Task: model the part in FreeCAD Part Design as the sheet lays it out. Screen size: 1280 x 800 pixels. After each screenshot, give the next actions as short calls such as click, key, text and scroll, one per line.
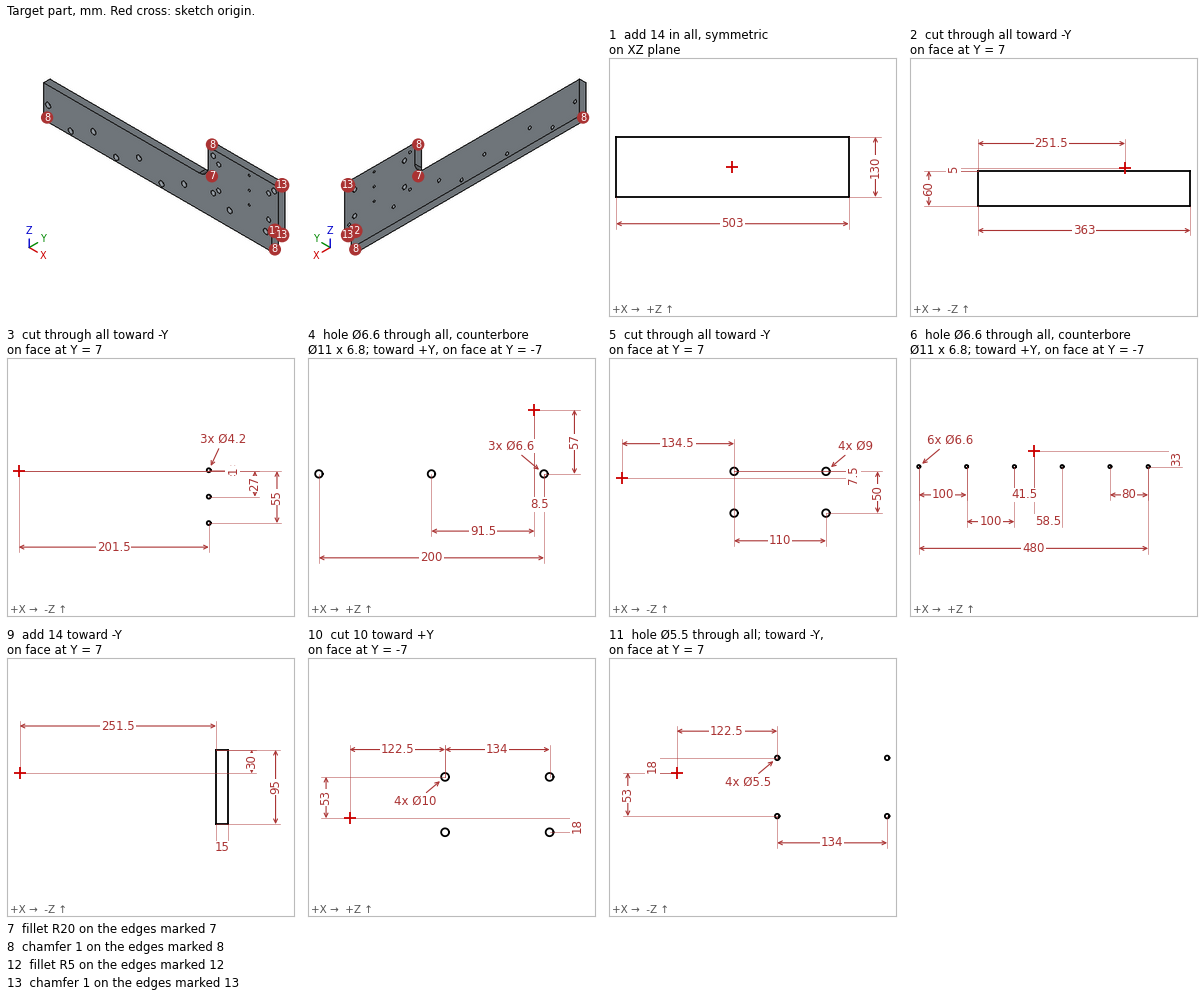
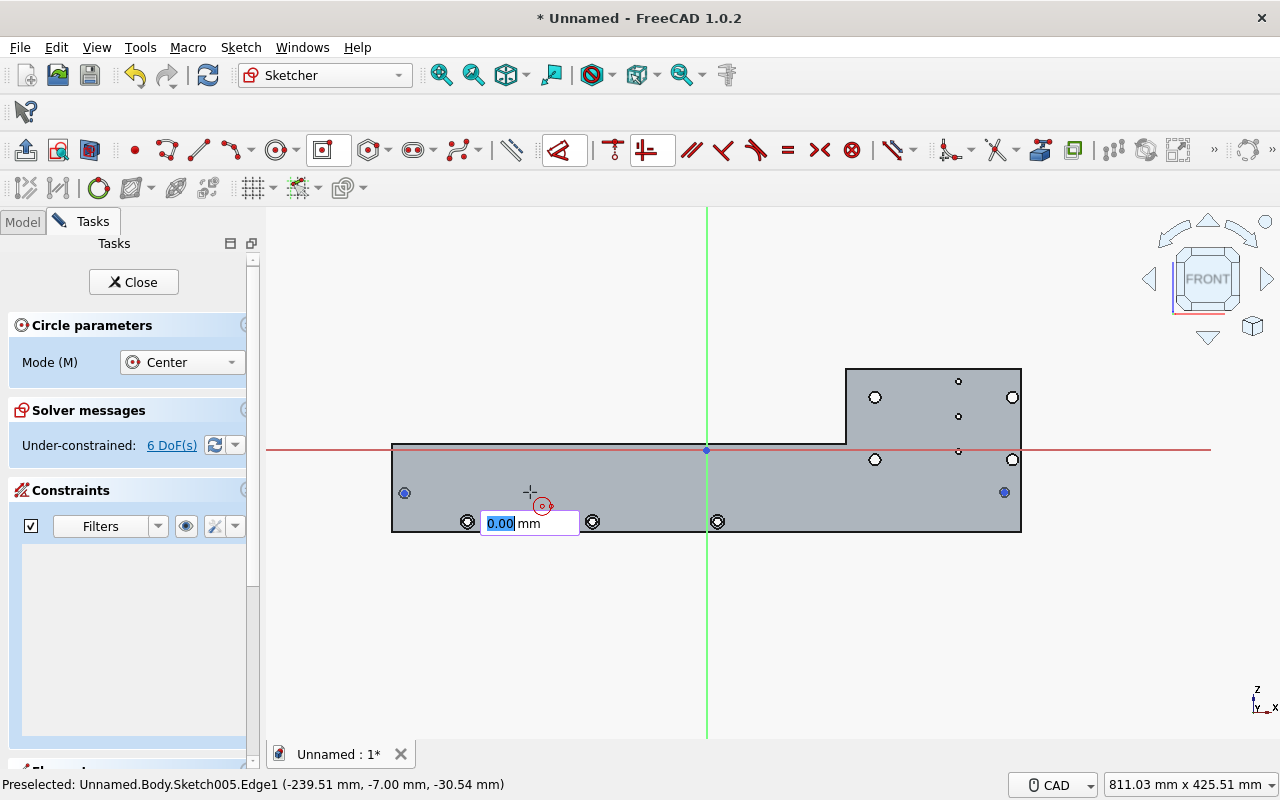
scroll(533, 489, up, 7)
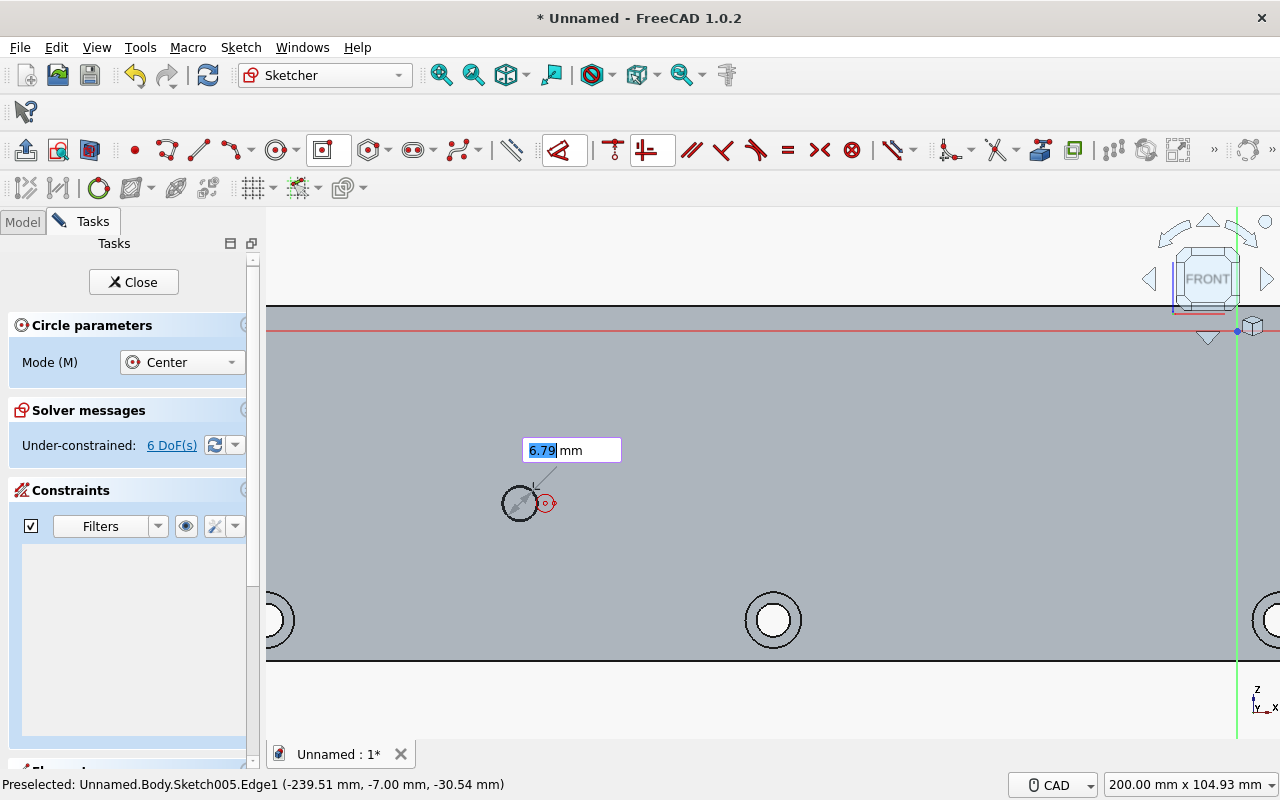
click(532, 487)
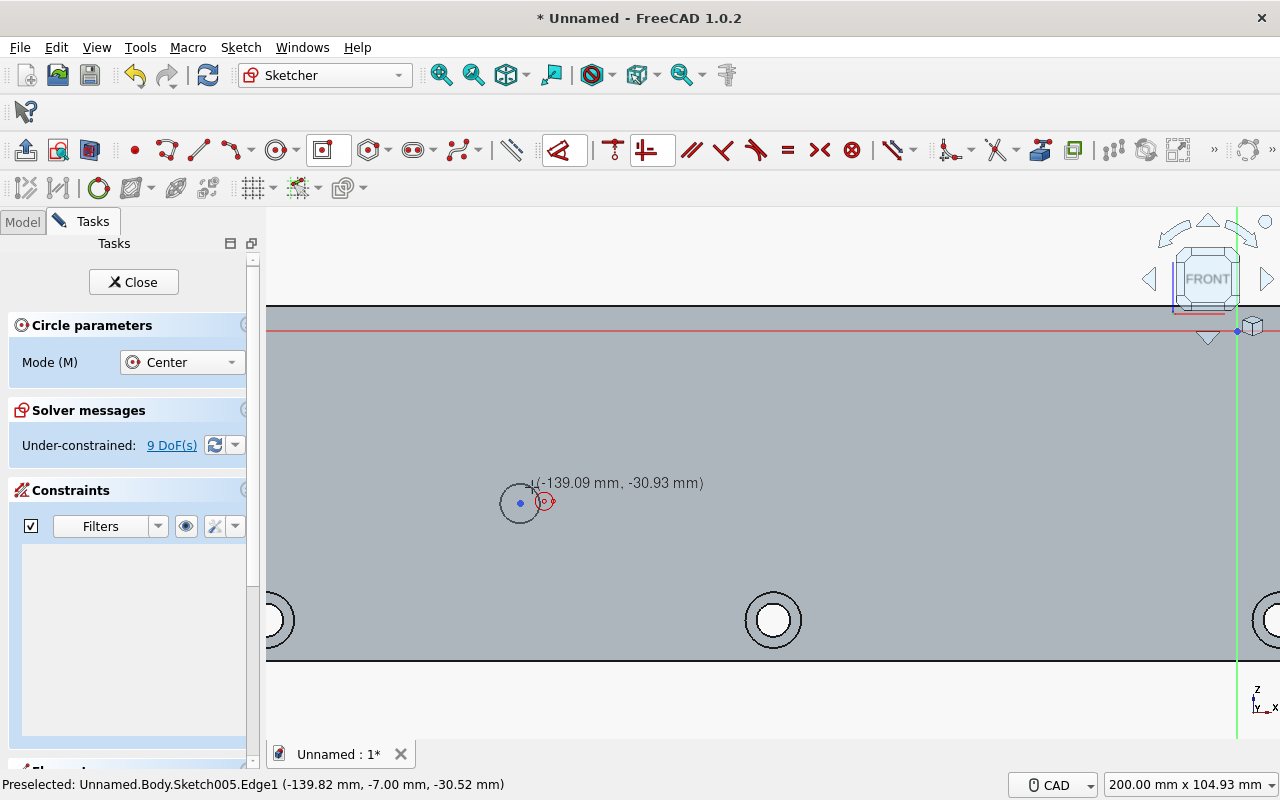
scroll(1027, 498, up, 2)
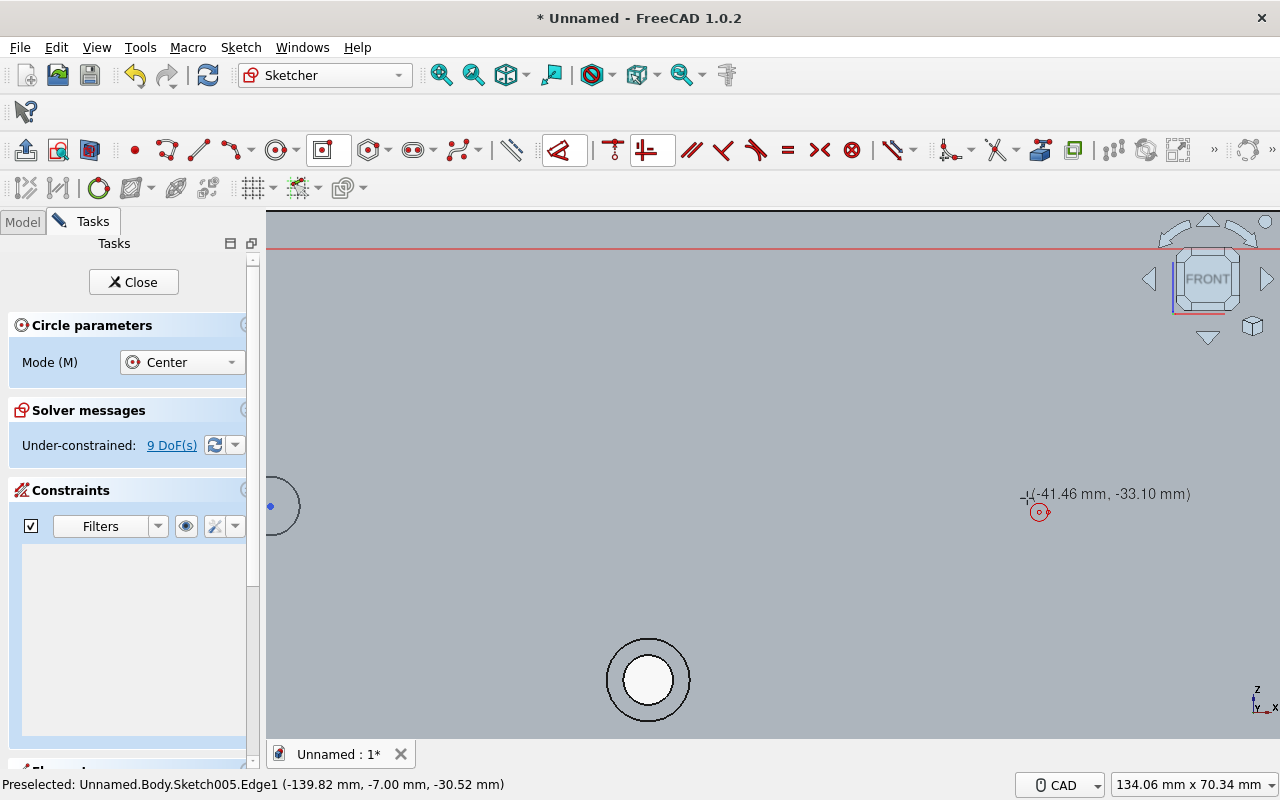
scroll(581, 490, down, 9)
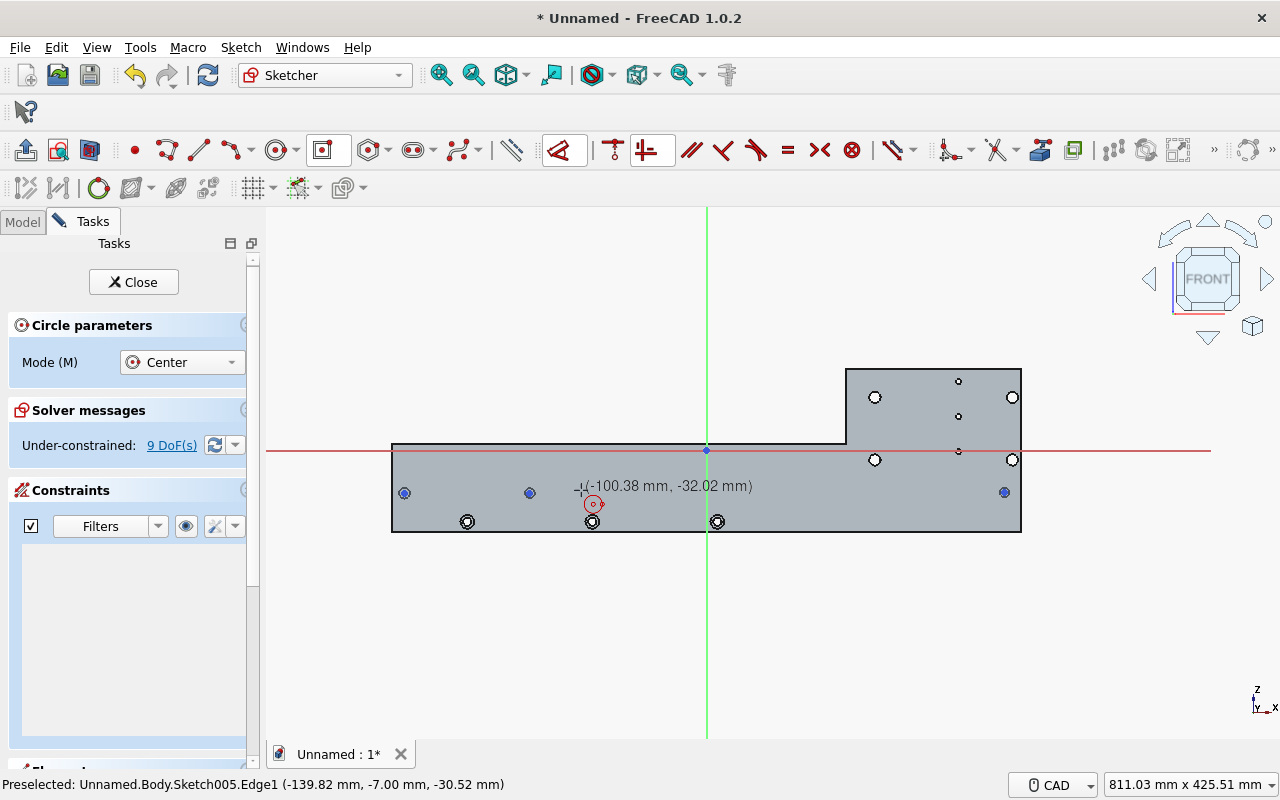
click(655, 492)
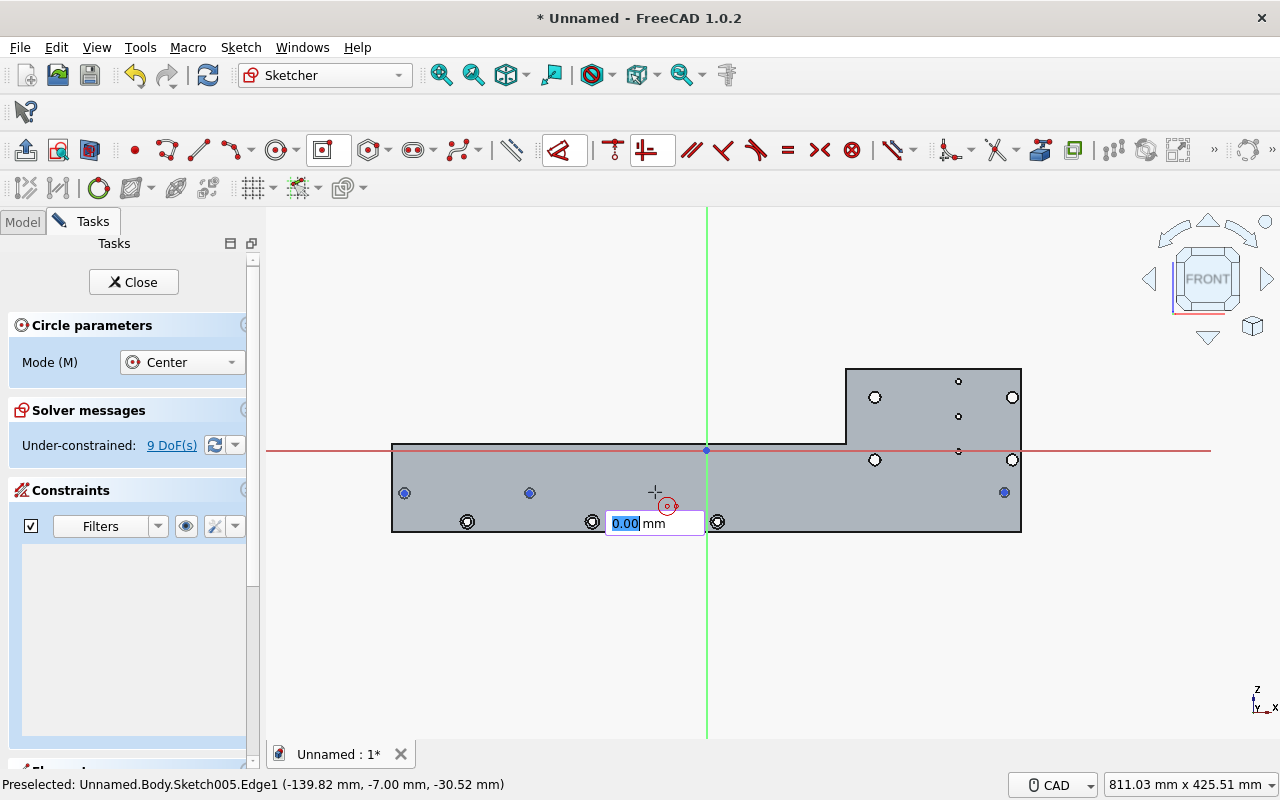
scroll(658, 489, up, 7)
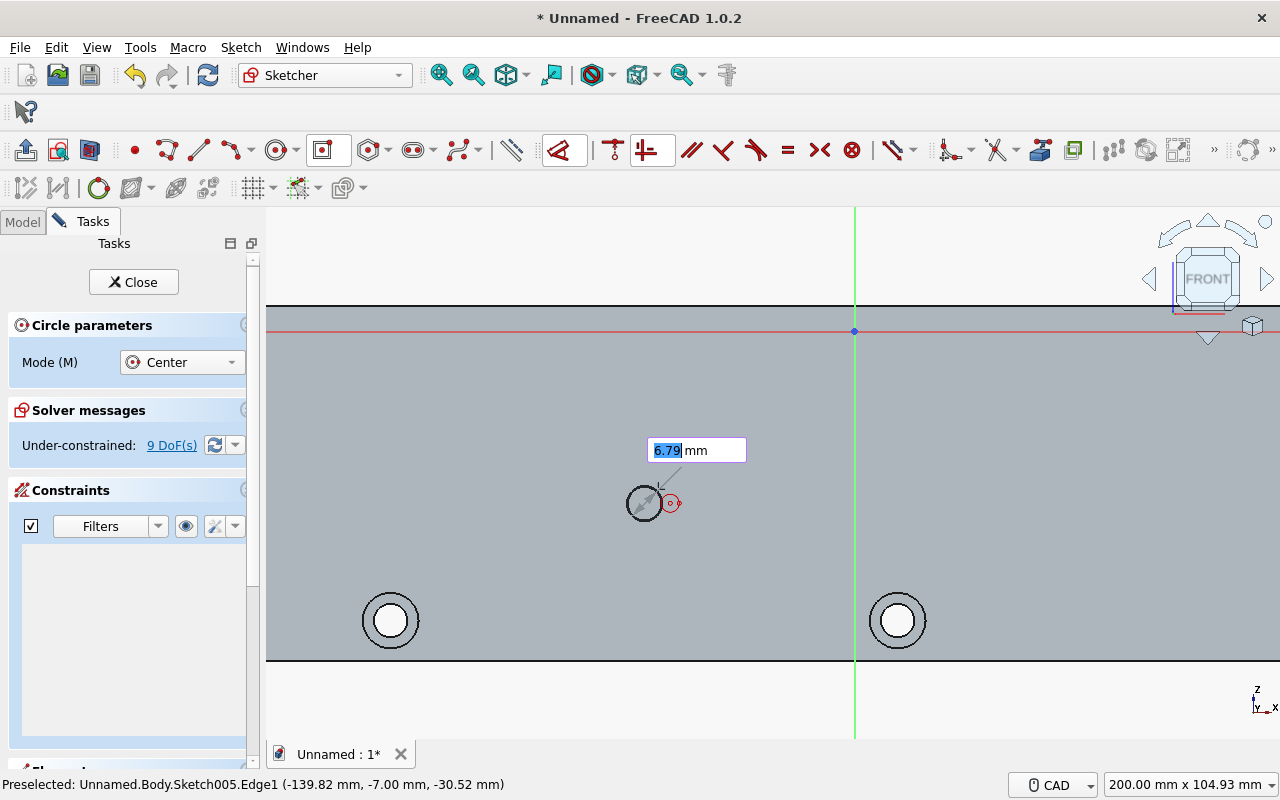
click(656, 487)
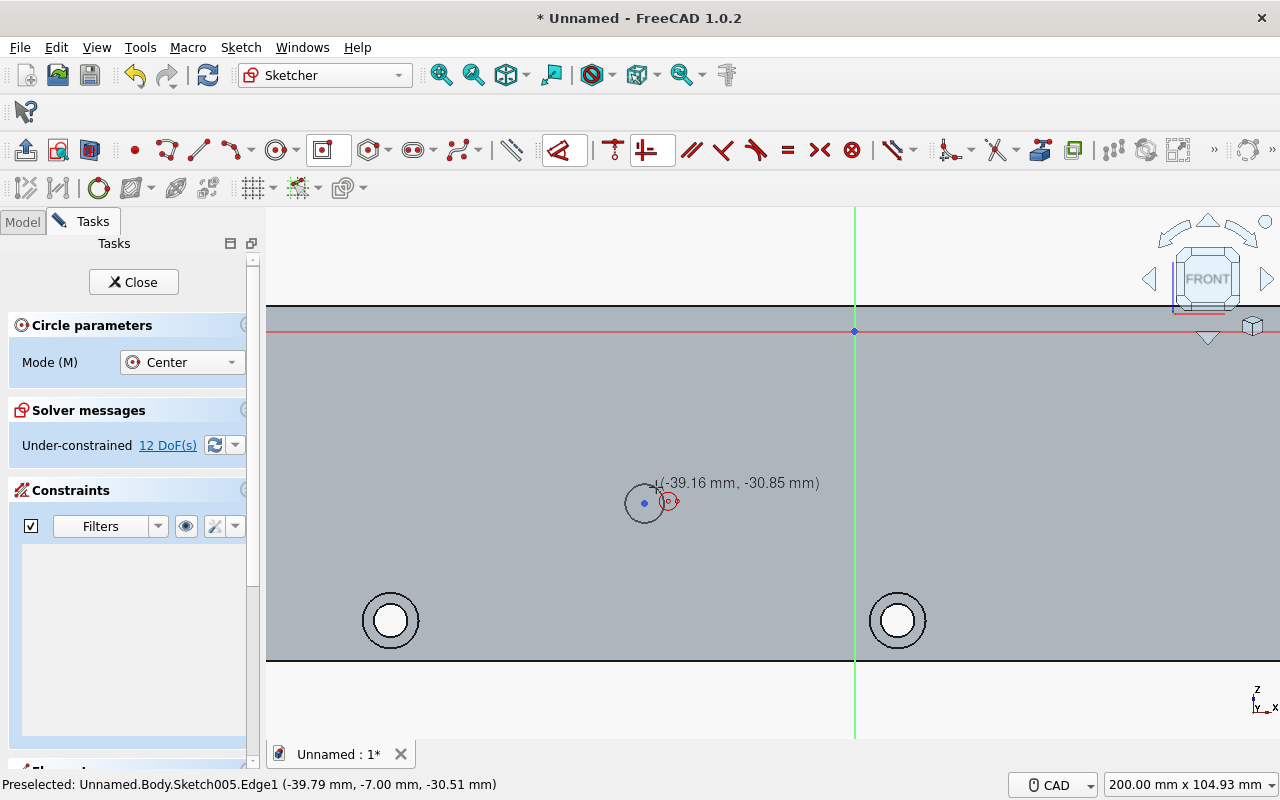
scroll(658, 489, down, 7)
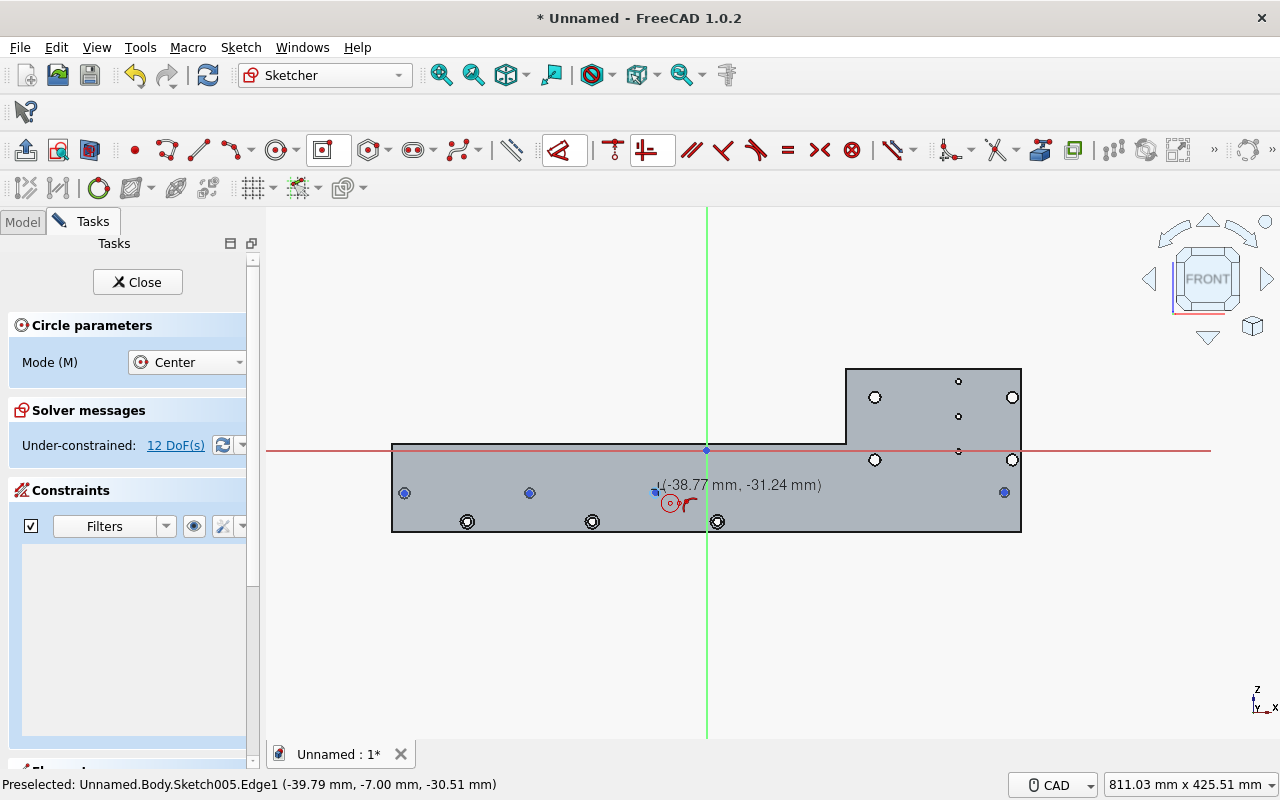
scroll(780, 492, up, 9)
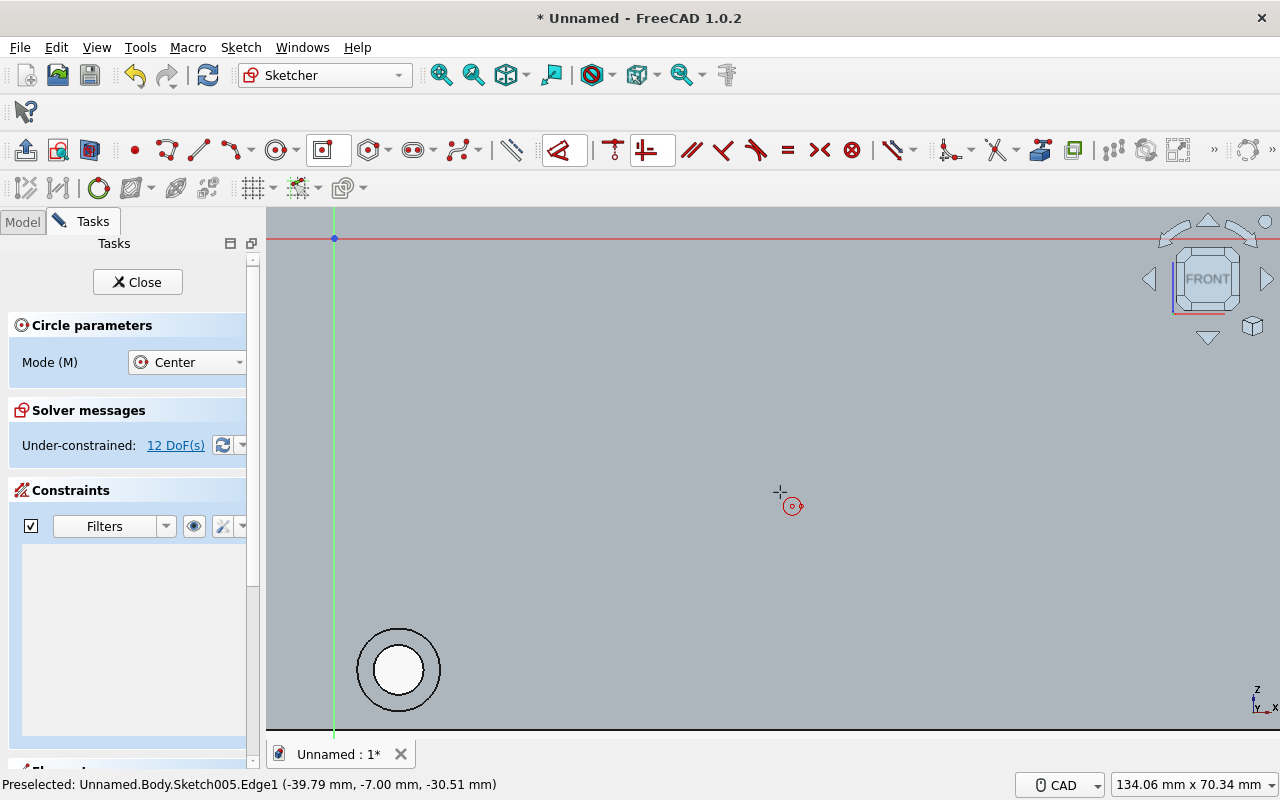
scroll(780, 492, down, 9)